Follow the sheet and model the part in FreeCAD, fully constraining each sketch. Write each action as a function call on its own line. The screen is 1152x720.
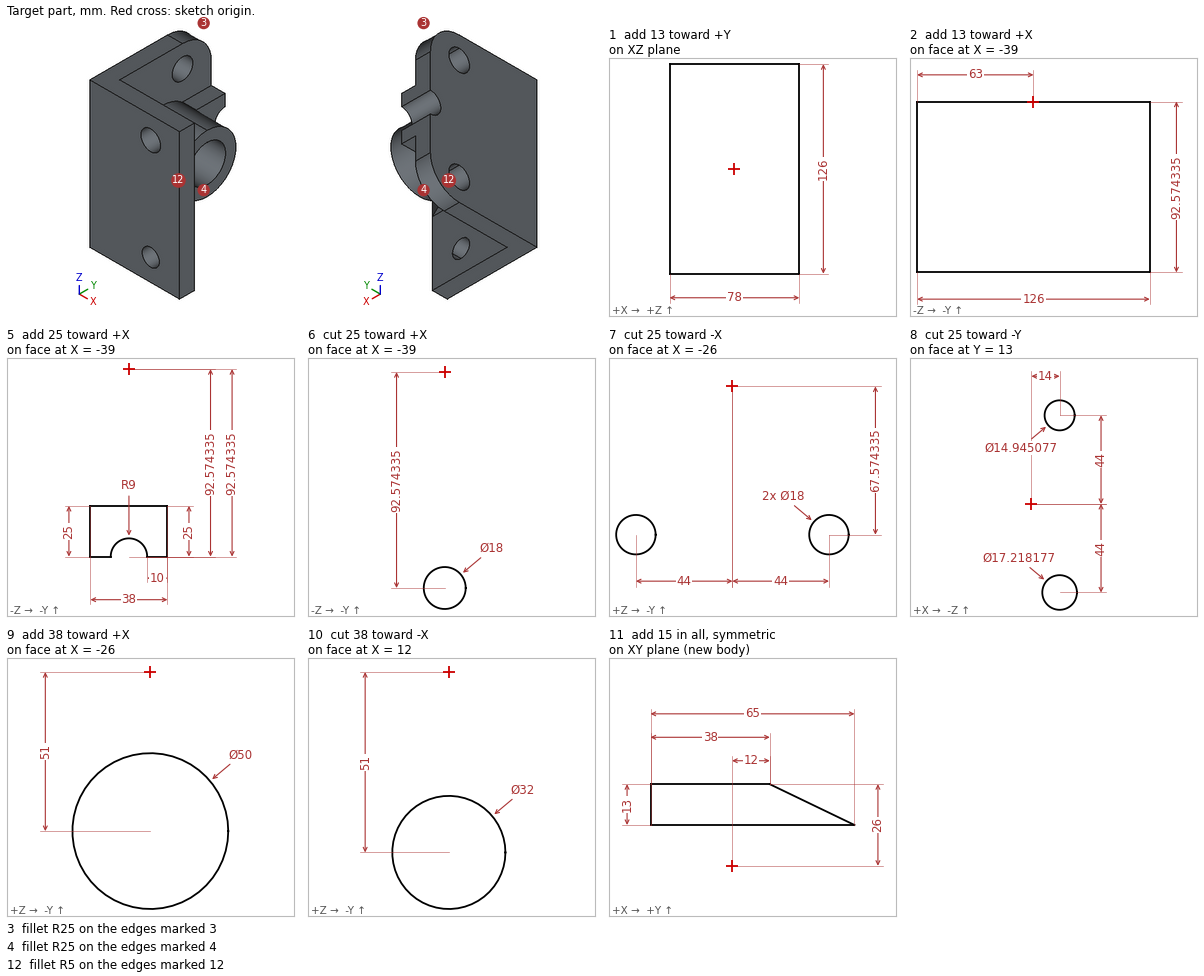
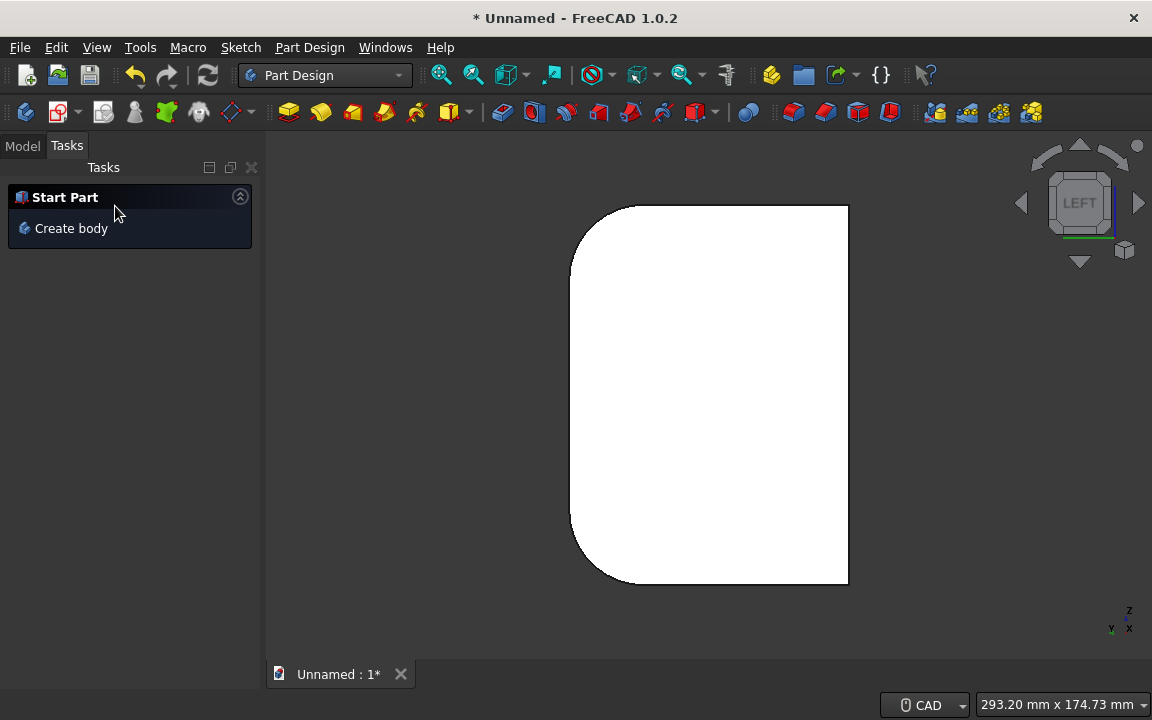
click(709, 394)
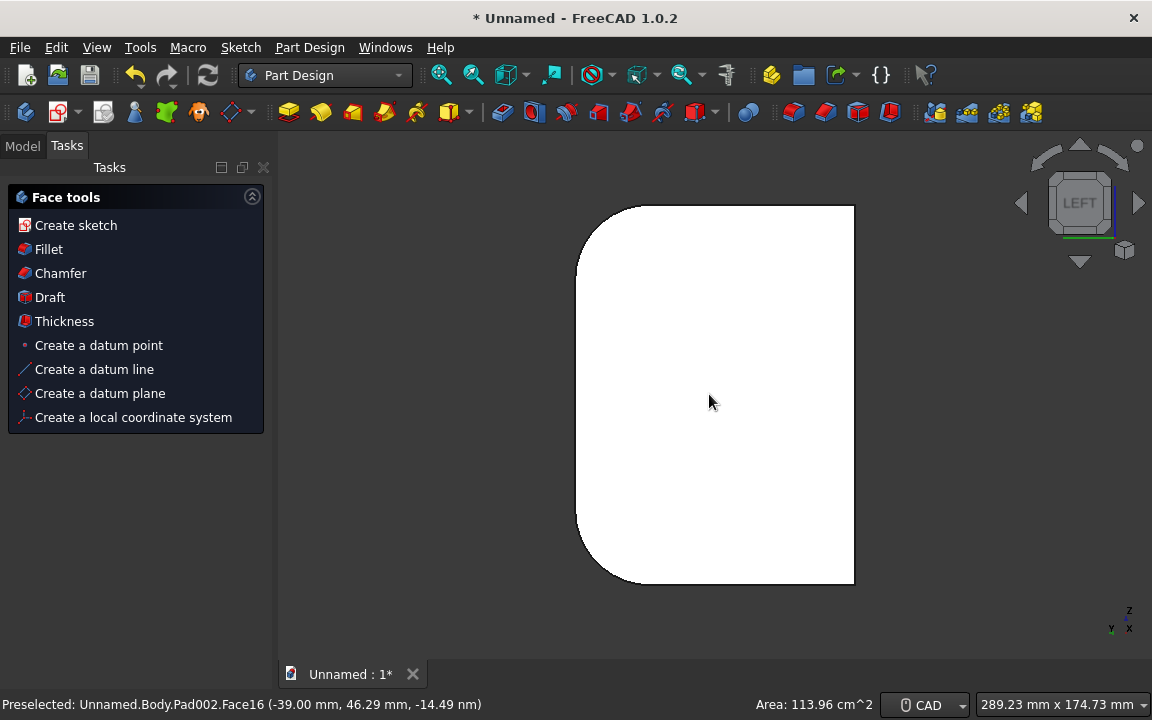
click(58, 112)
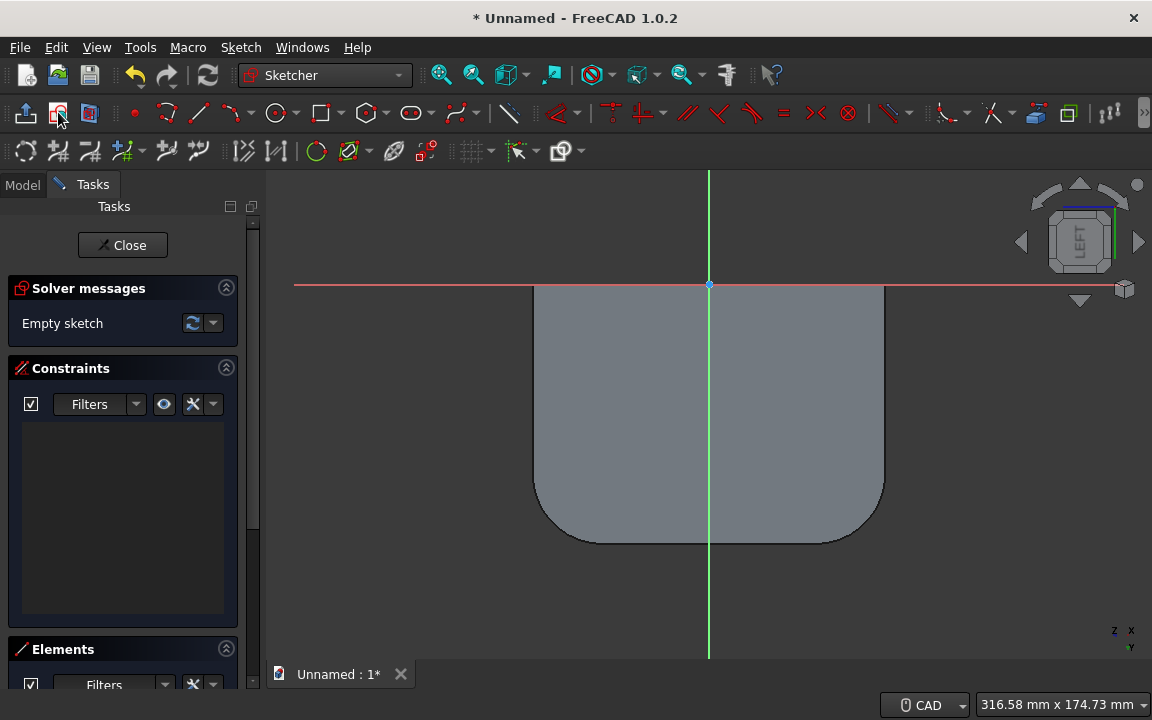
scroll(723, 570, up, 9)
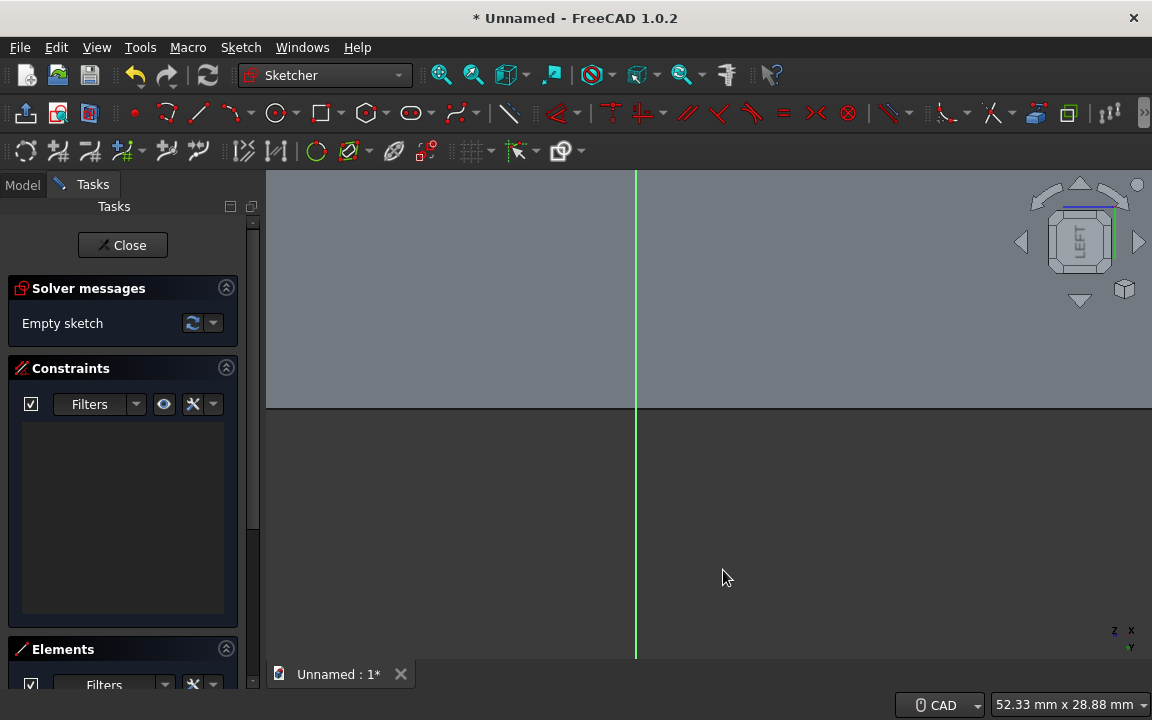
key(g)
key(c)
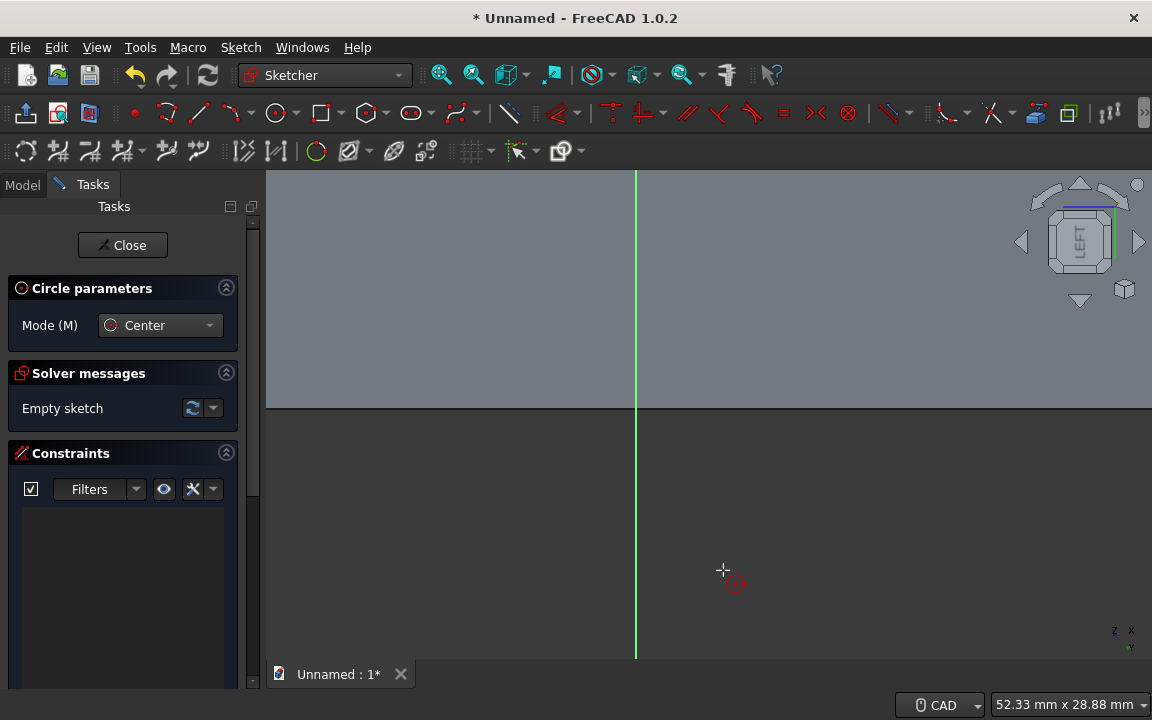
click(636, 409)
move(743, 301)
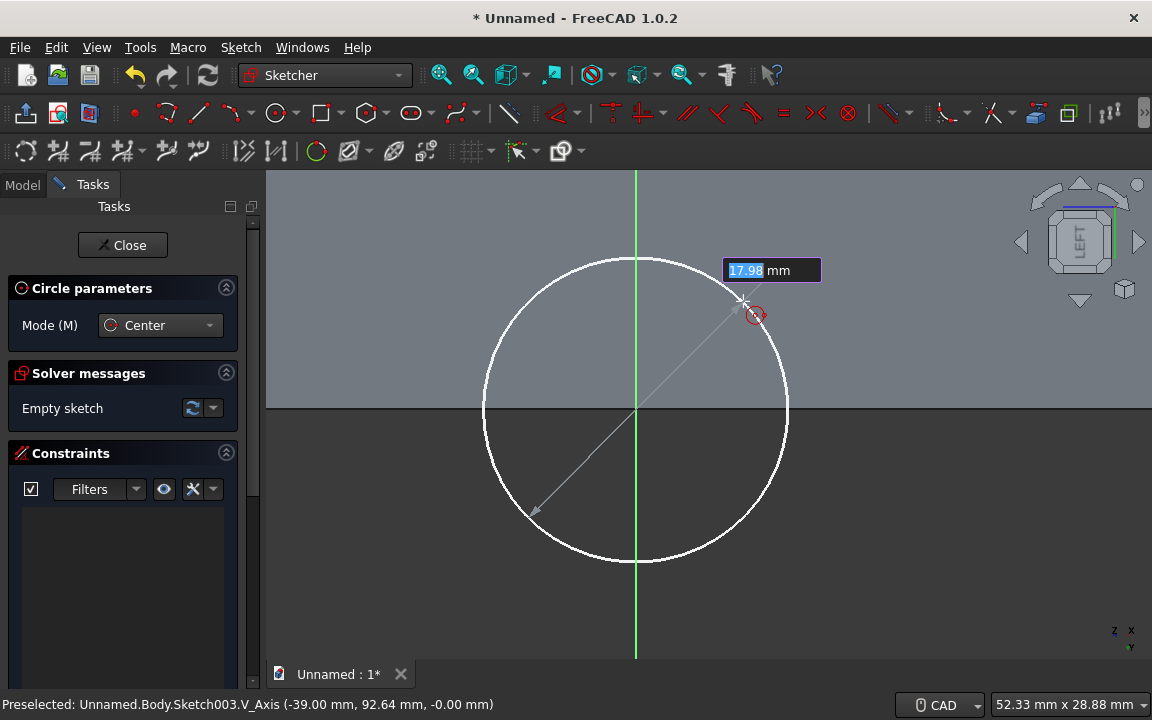
text(18)
key(Return)
key(Escape)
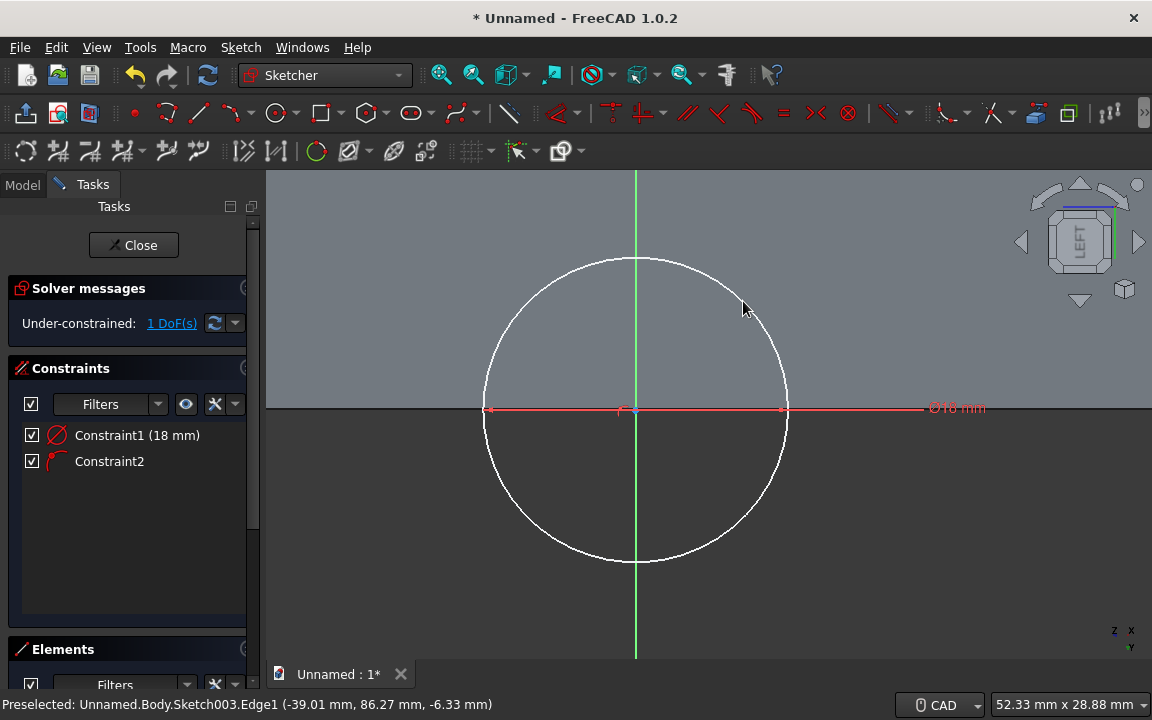
click(636, 410)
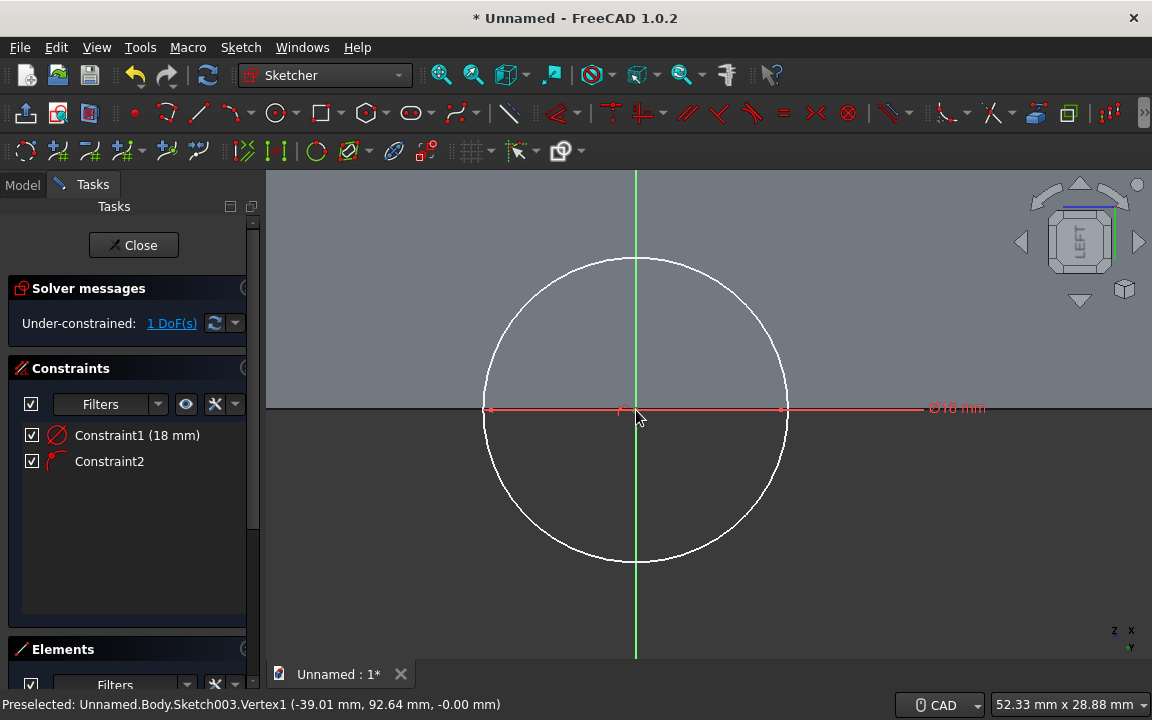
key(i)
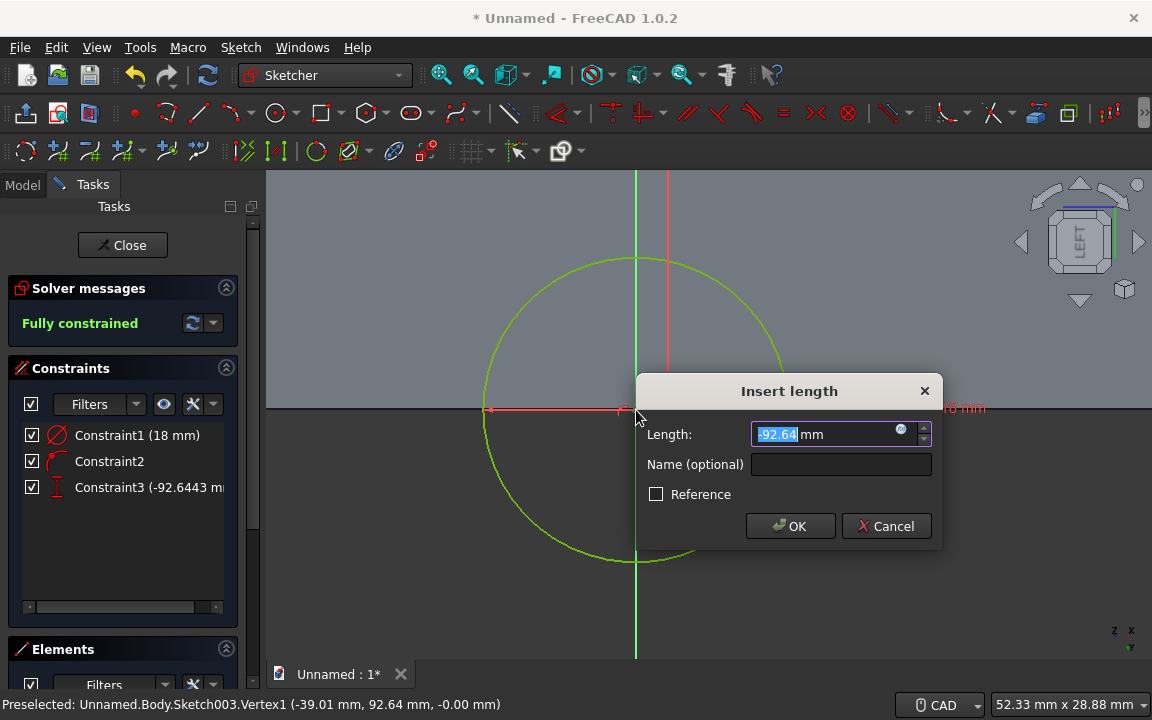
text(-92.574335)
key(Return)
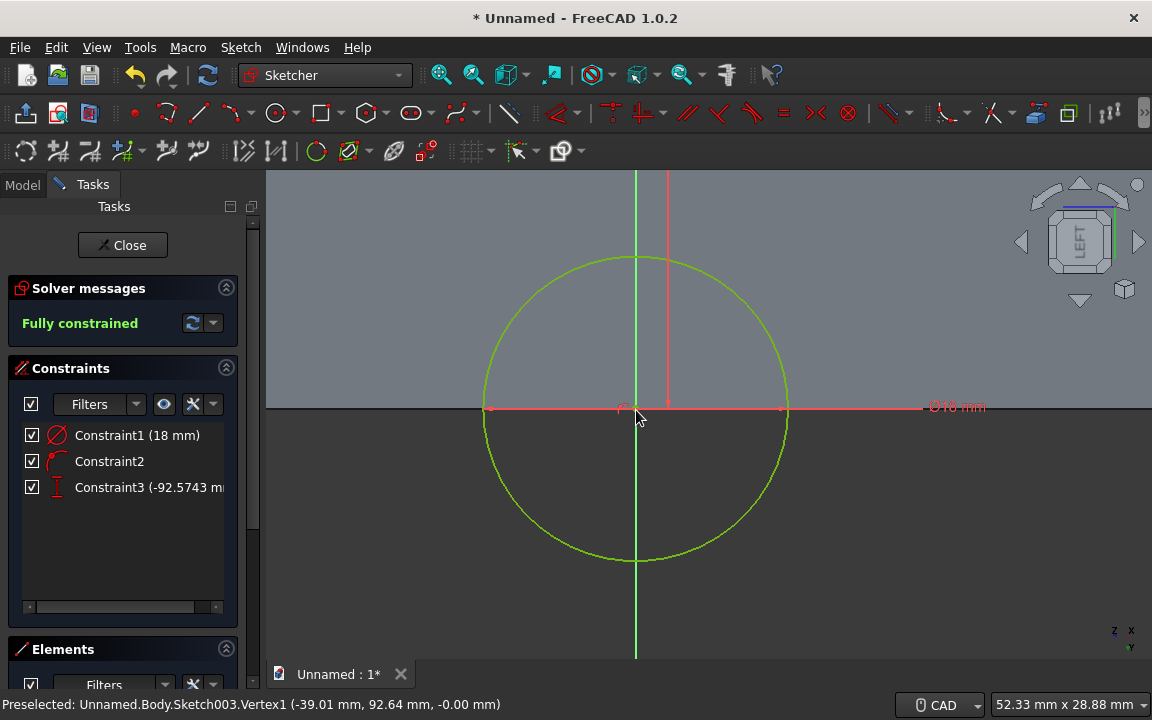
click(123, 245)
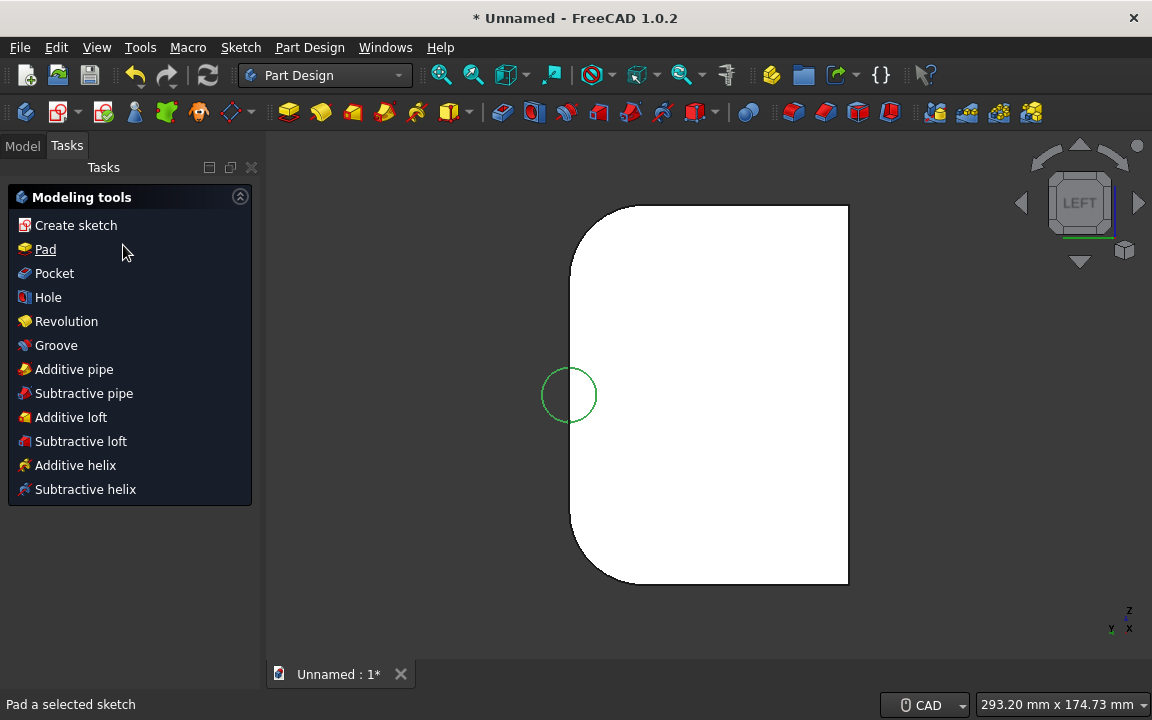
click(504, 112)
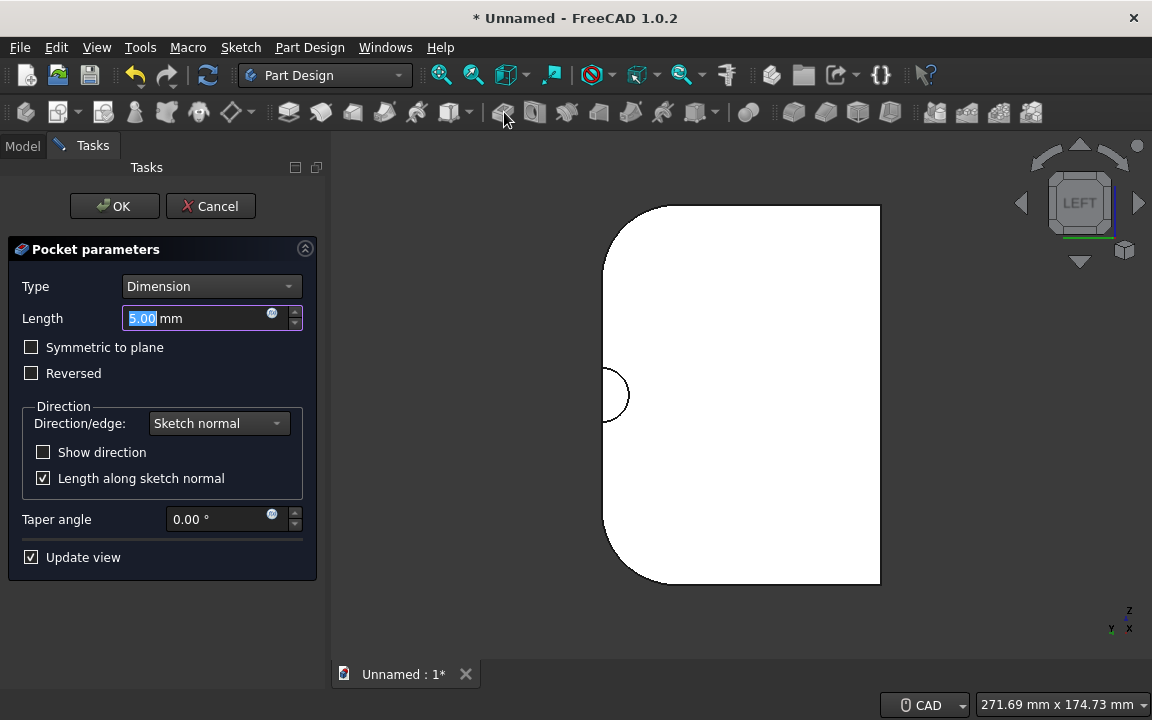
text(25)
key(Tab)